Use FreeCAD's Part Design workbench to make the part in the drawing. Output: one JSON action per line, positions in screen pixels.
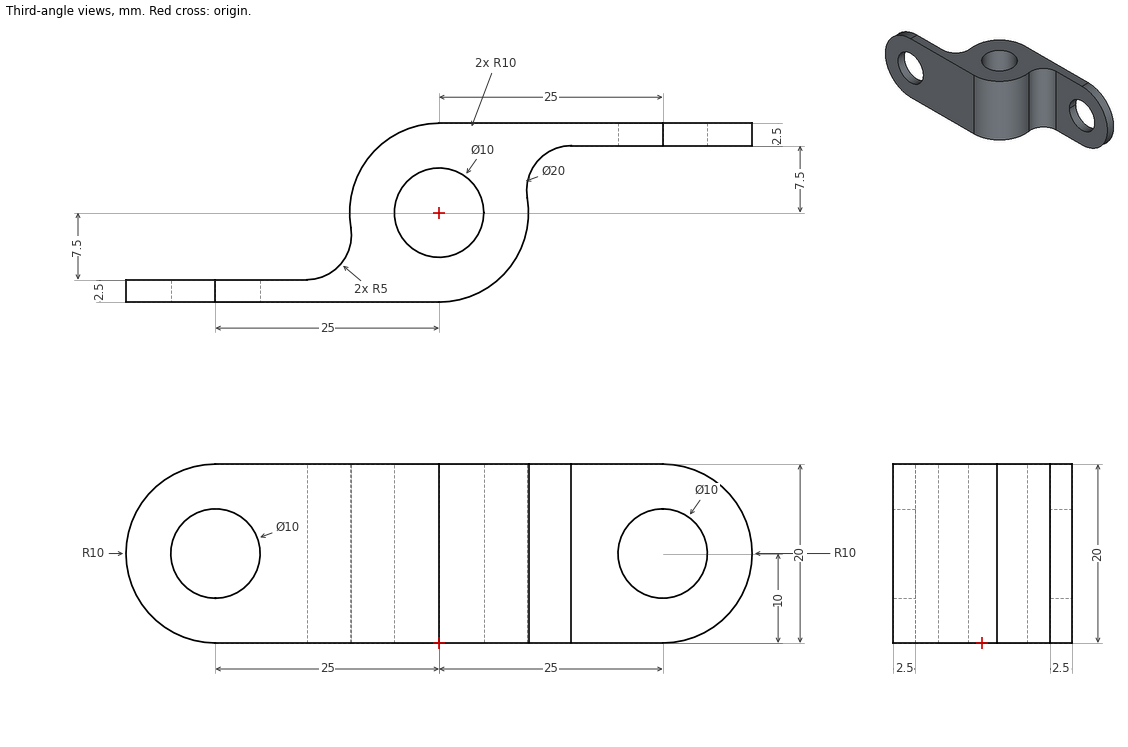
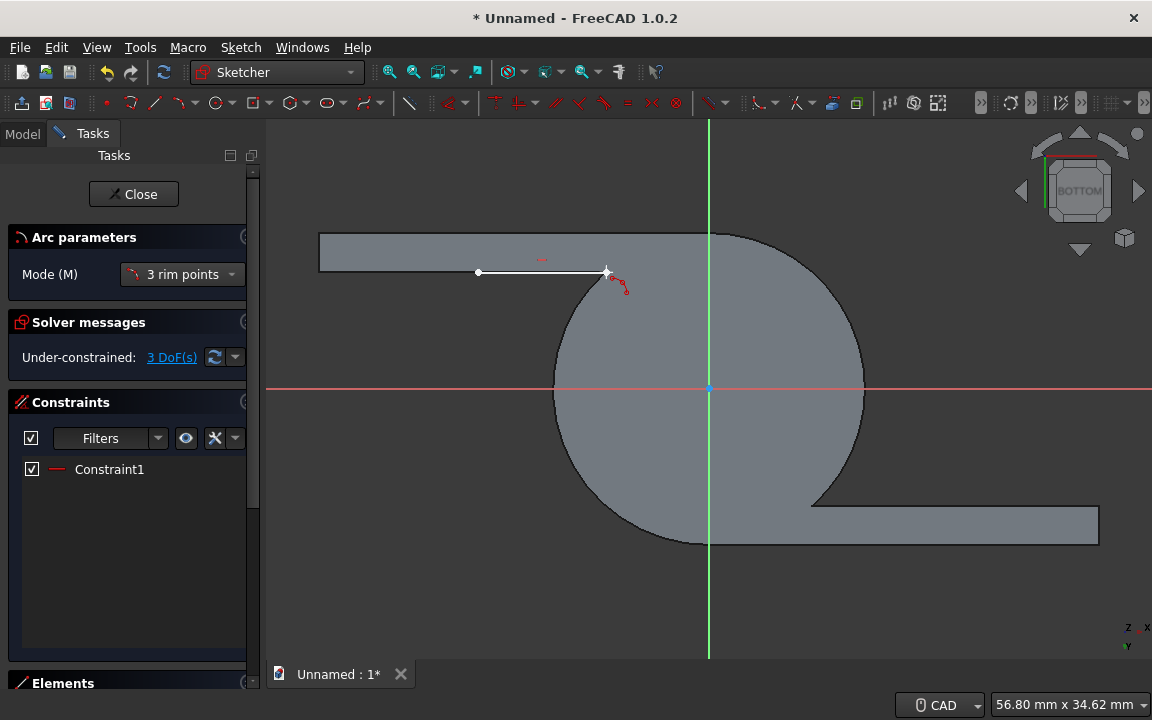
{"action": "left_click", "coordinate": [606, 273]}
{"action": "left_click", "coordinate": [555, 363]}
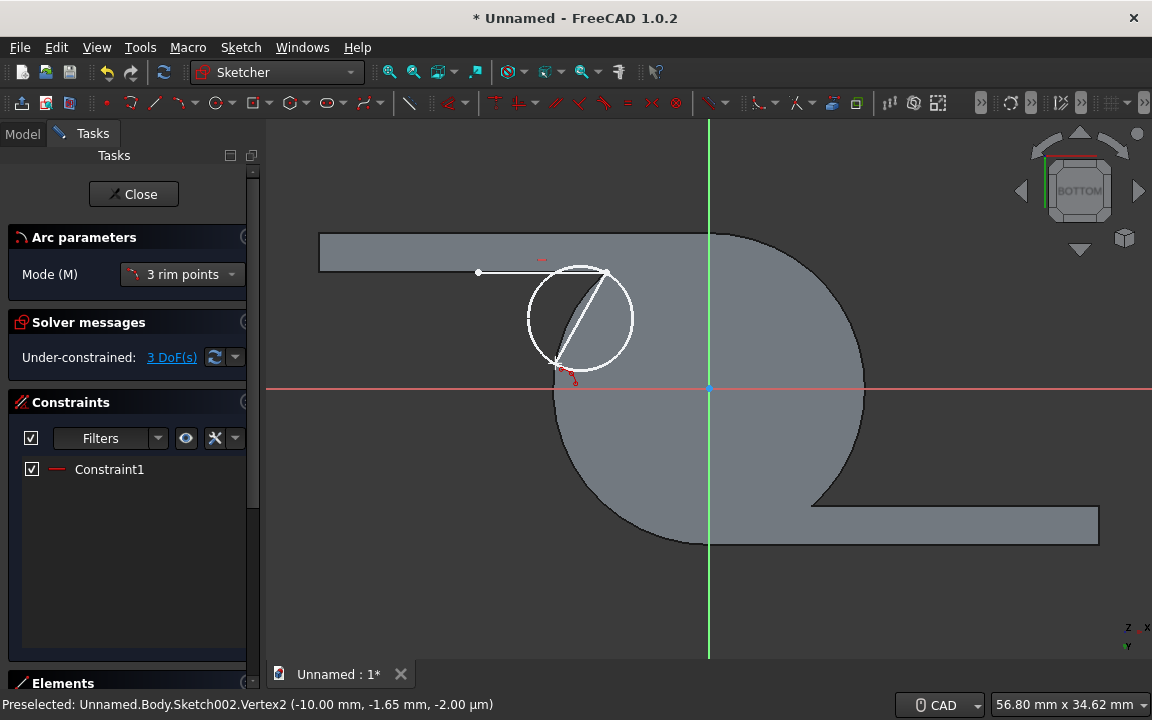
{"action": "scroll", "coordinate": [573, 313], "scroll_direction": "up", "scroll_amount": 3}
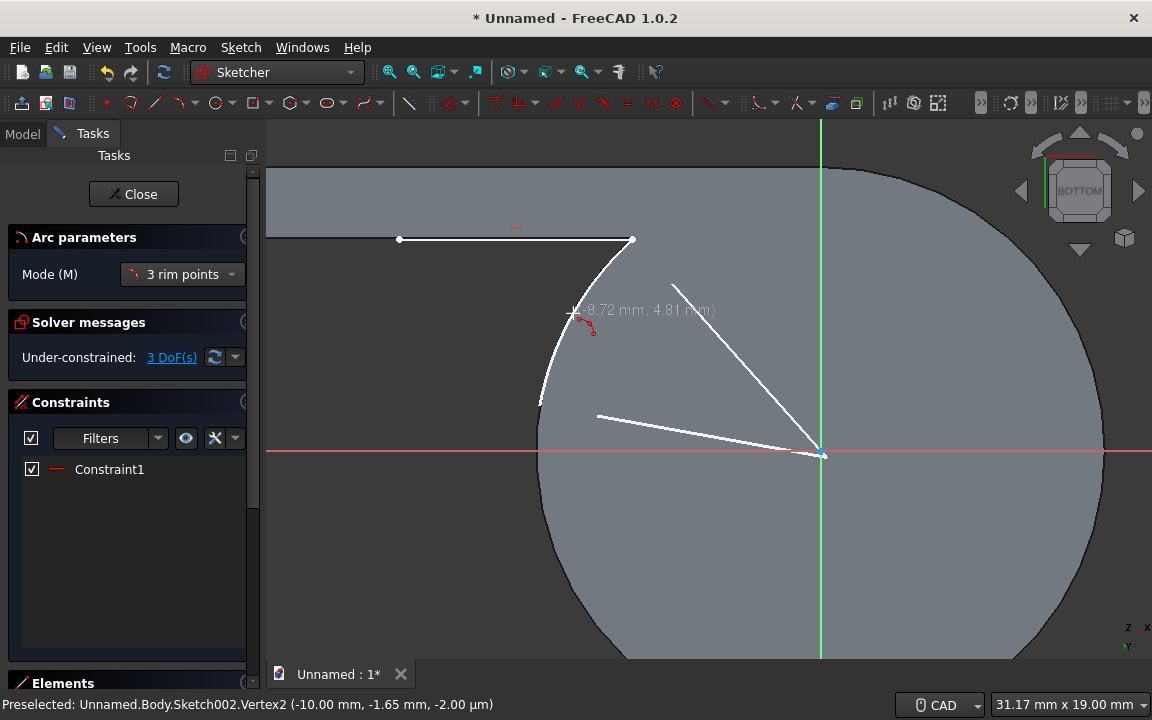
{"action": "left_click", "coordinate": [572, 313]}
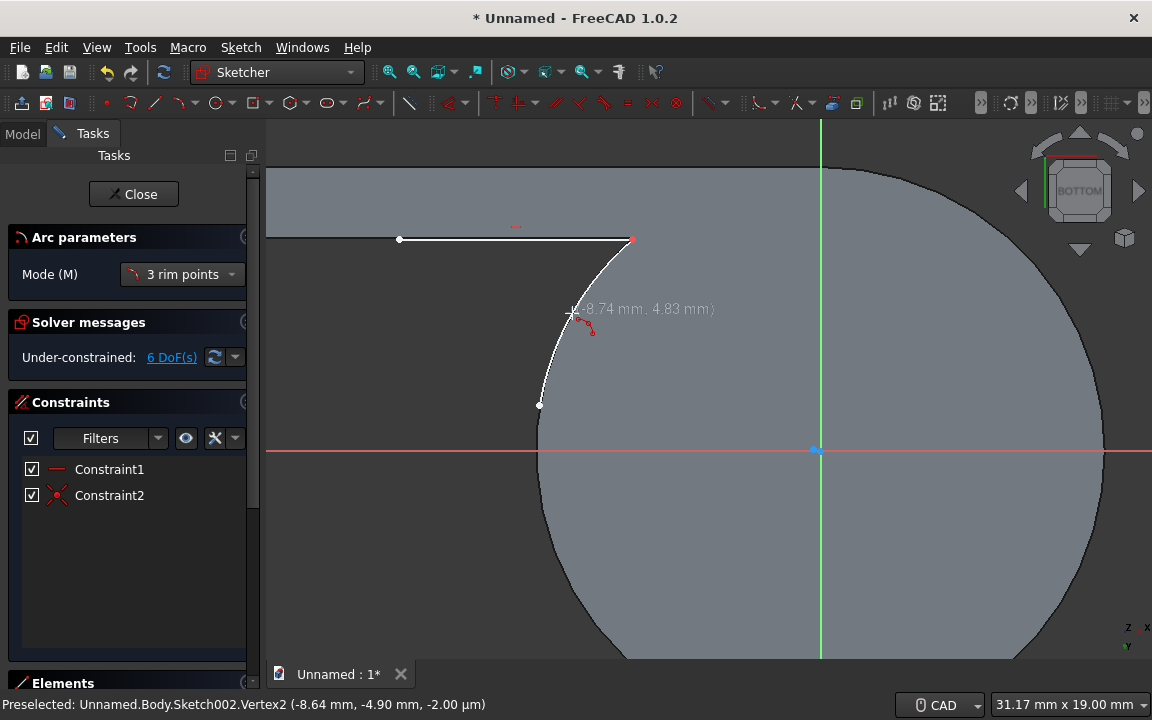
{"action": "left_click", "coordinate": [540, 406]}
{"action": "left_click", "coordinate": [400, 240]}
{"action": "left_click", "coordinate": [509, 288]}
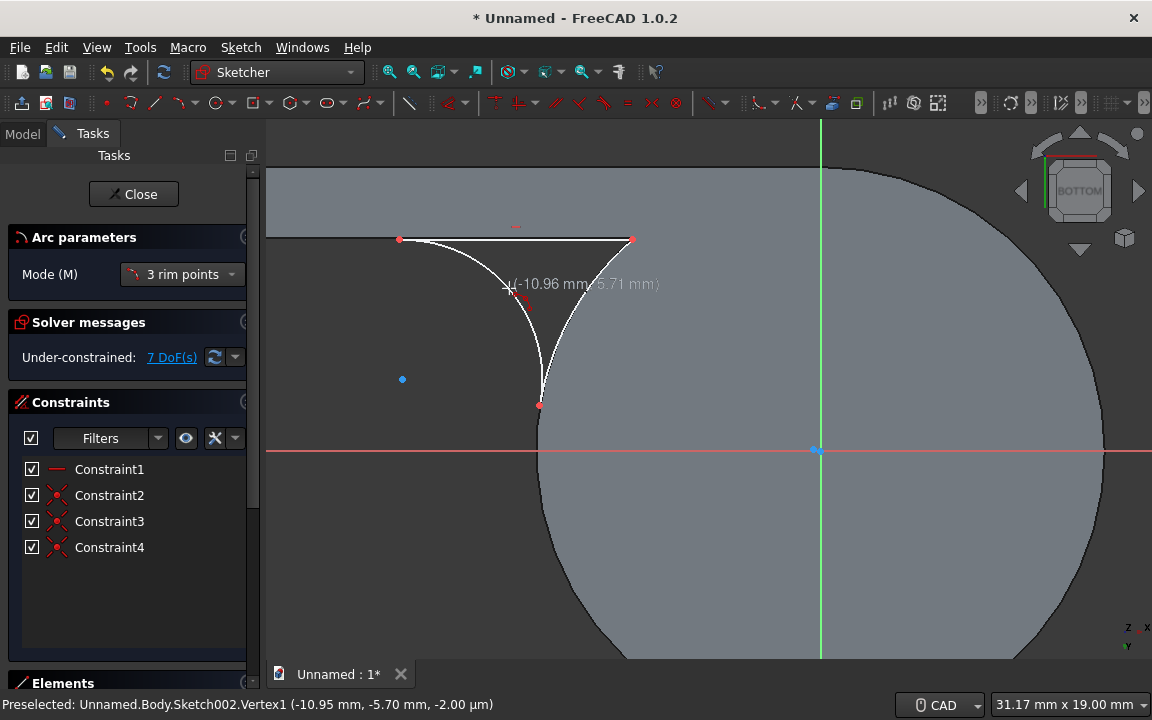
{"action": "key", "text": "g l"}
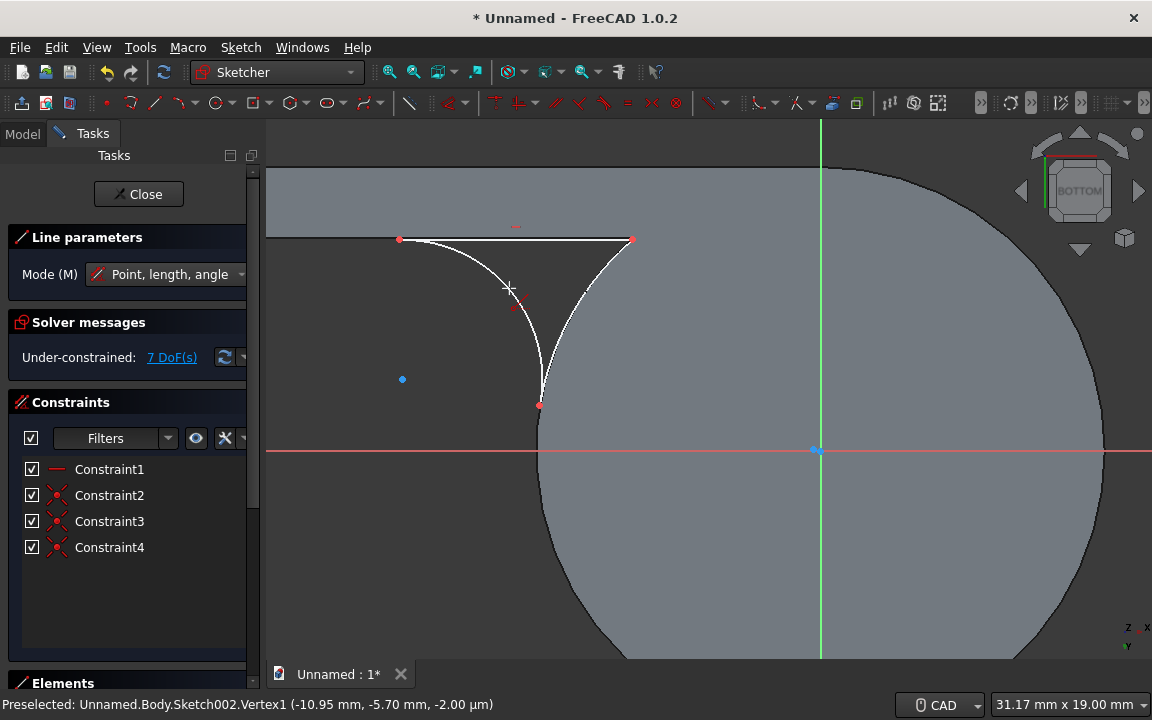
{"action": "scroll", "coordinate": [422, 313], "scroll_direction": "down", "scroll_amount": 3}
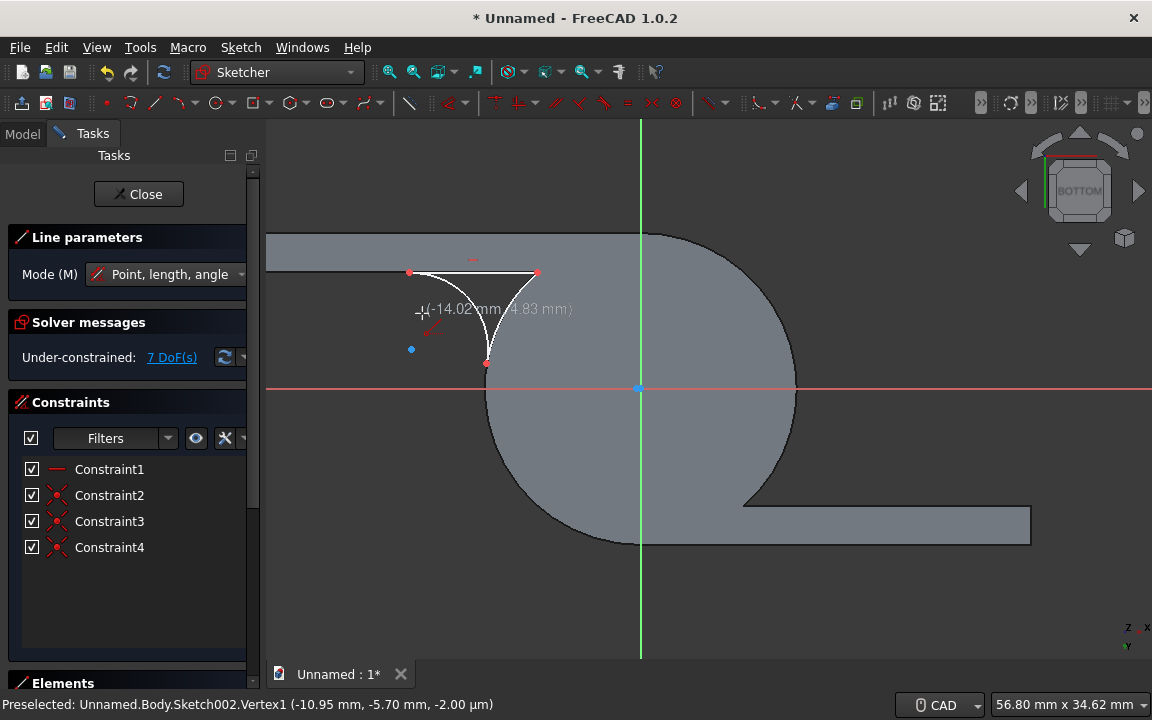
{"action": "left_click", "coordinate": [872, 506]}
{"action": "left_click", "coordinate": [744, 506]}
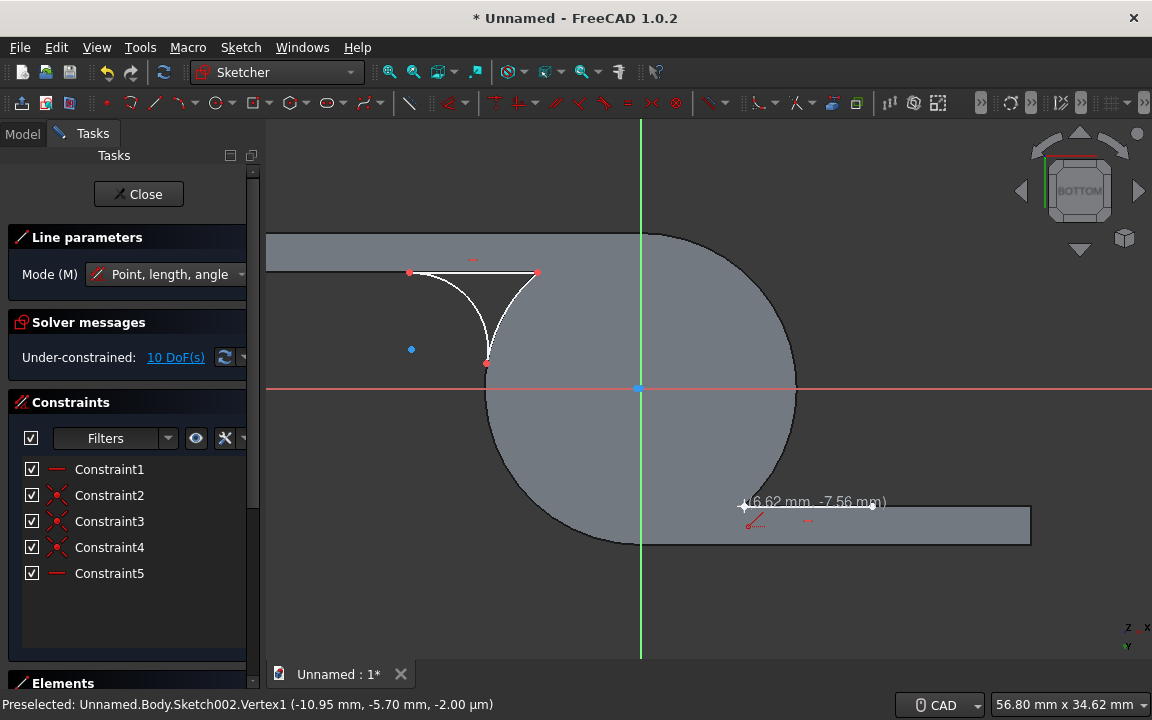
{"action": "key", "text": "g 3 a"}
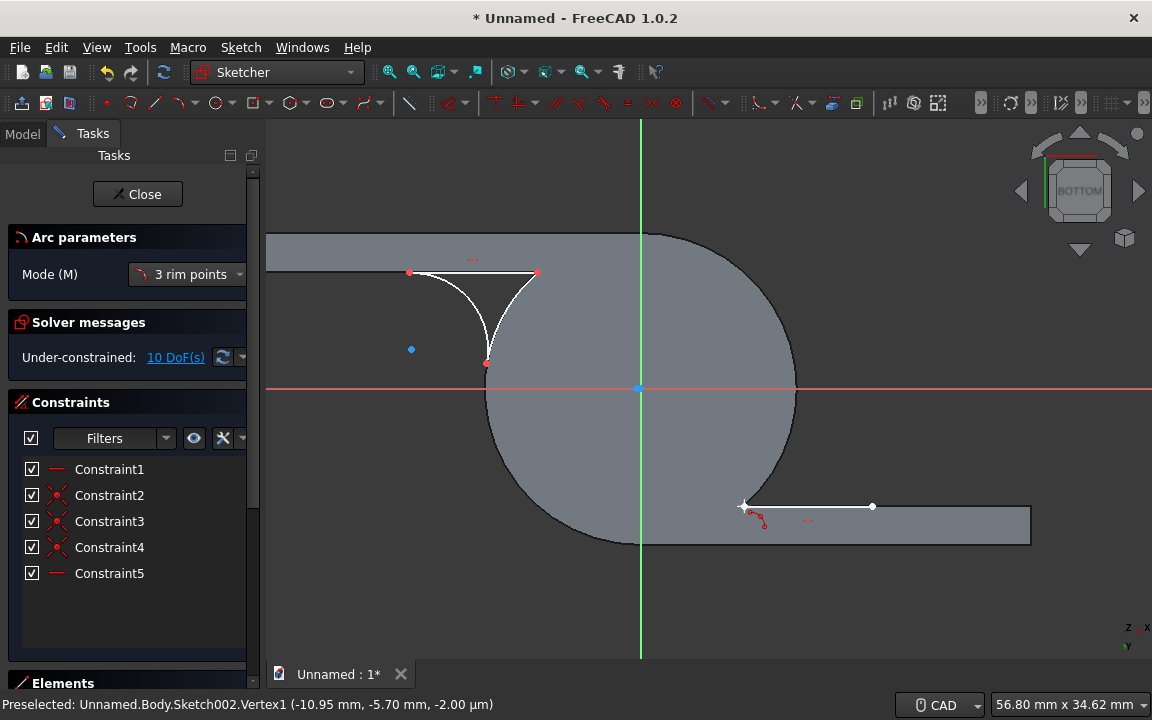
{"action": "left_click", "coordinate": [744, 507]}
{"action": "left_click", "coordinate": [795, 415]}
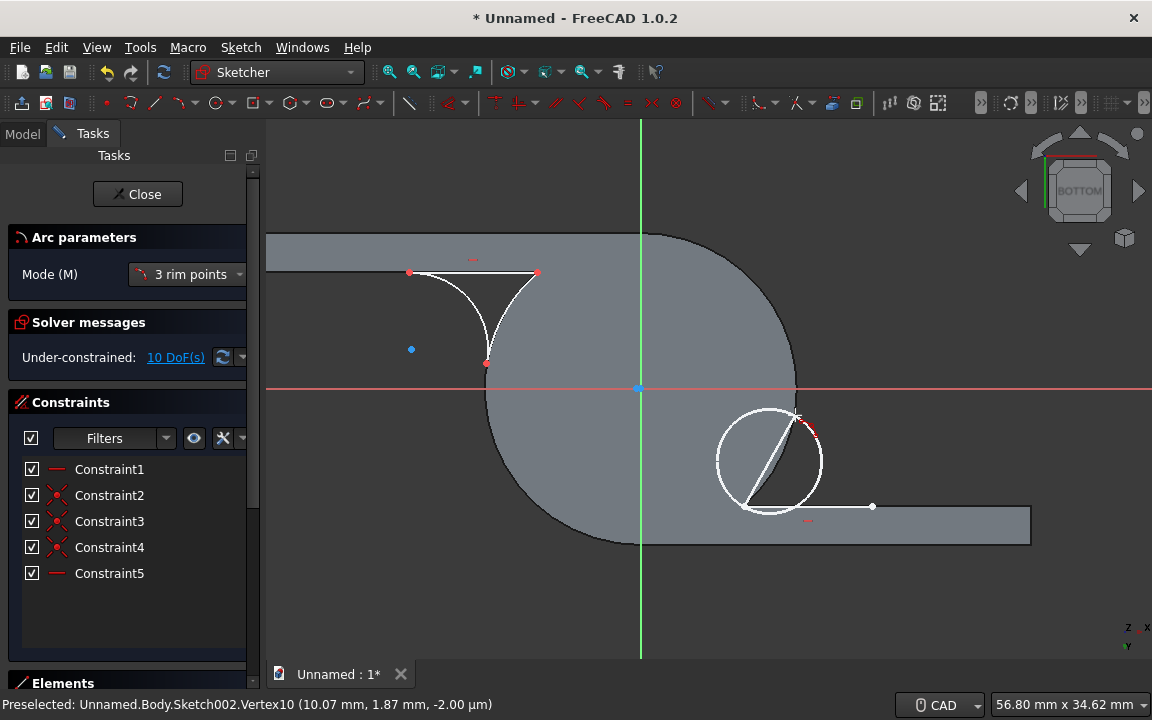
{"action": "scroll", "coordinate": [777, 465], "scroll_direction": "up", "scroll_amount": 3}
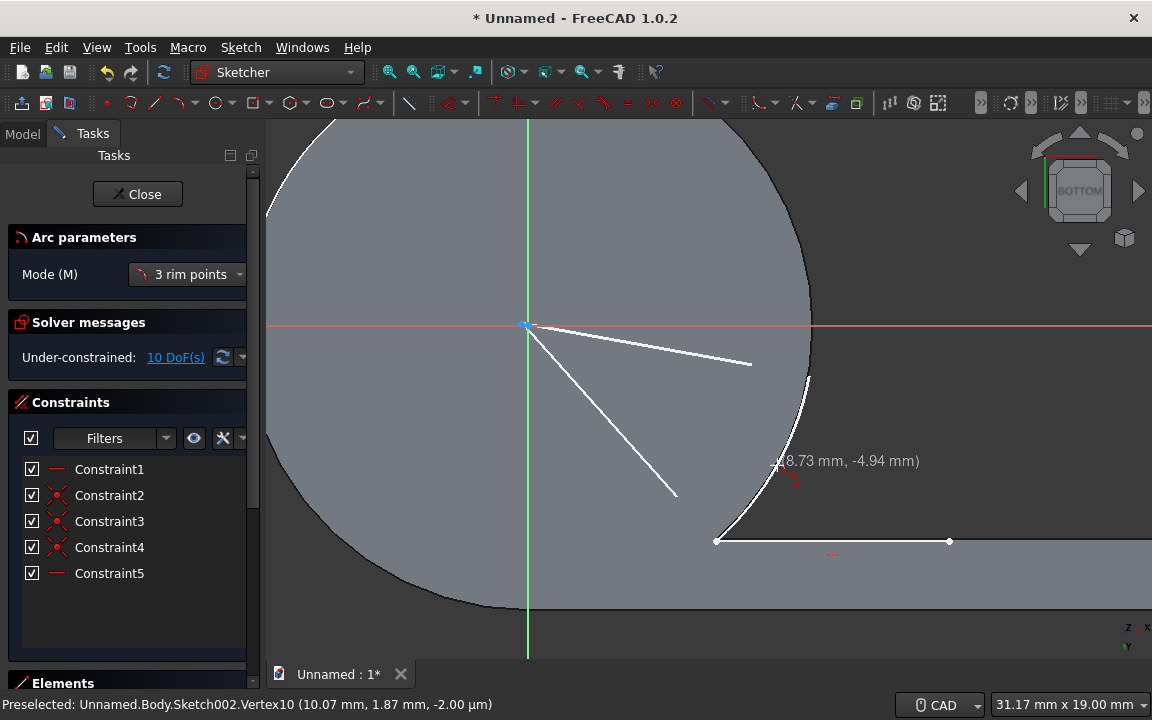
{"action": "left_click", "coordinate": [777, 464]}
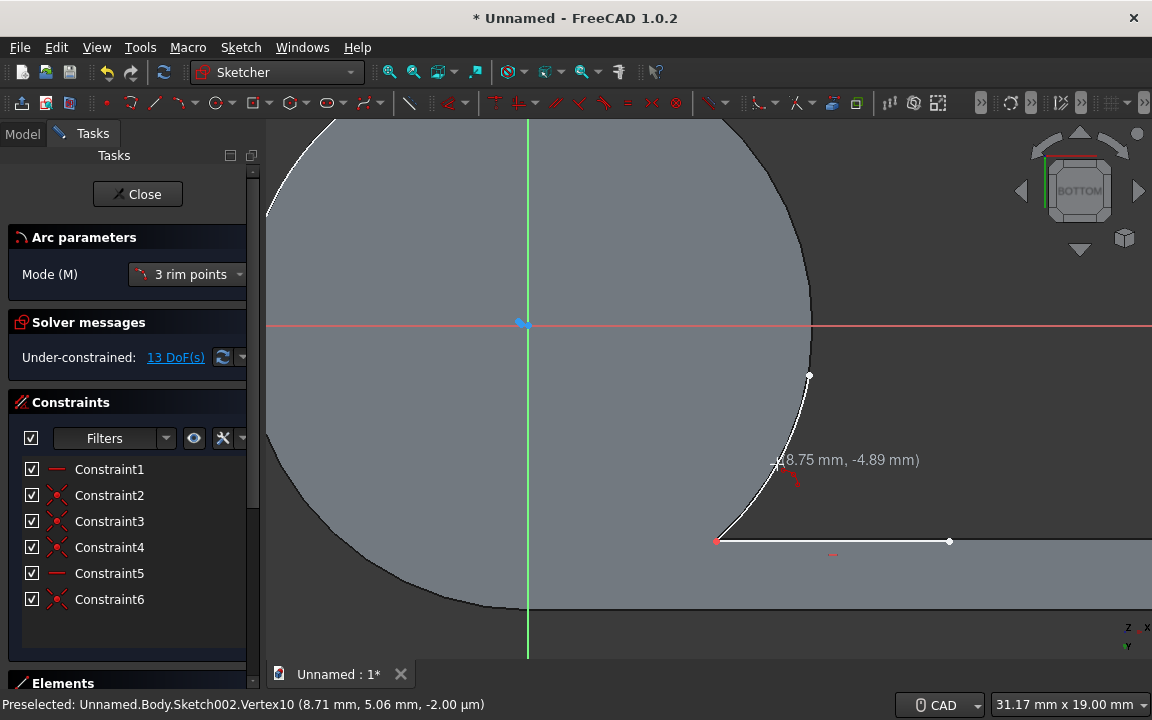
{"action": "left_click", "coordinate": [809, 375]}
{"action": "left_click", "coordinate": [950, 541]}
{"action": "left_click", "coordinate": [840, 489]}
{"action": "key", "text": "Escape"}